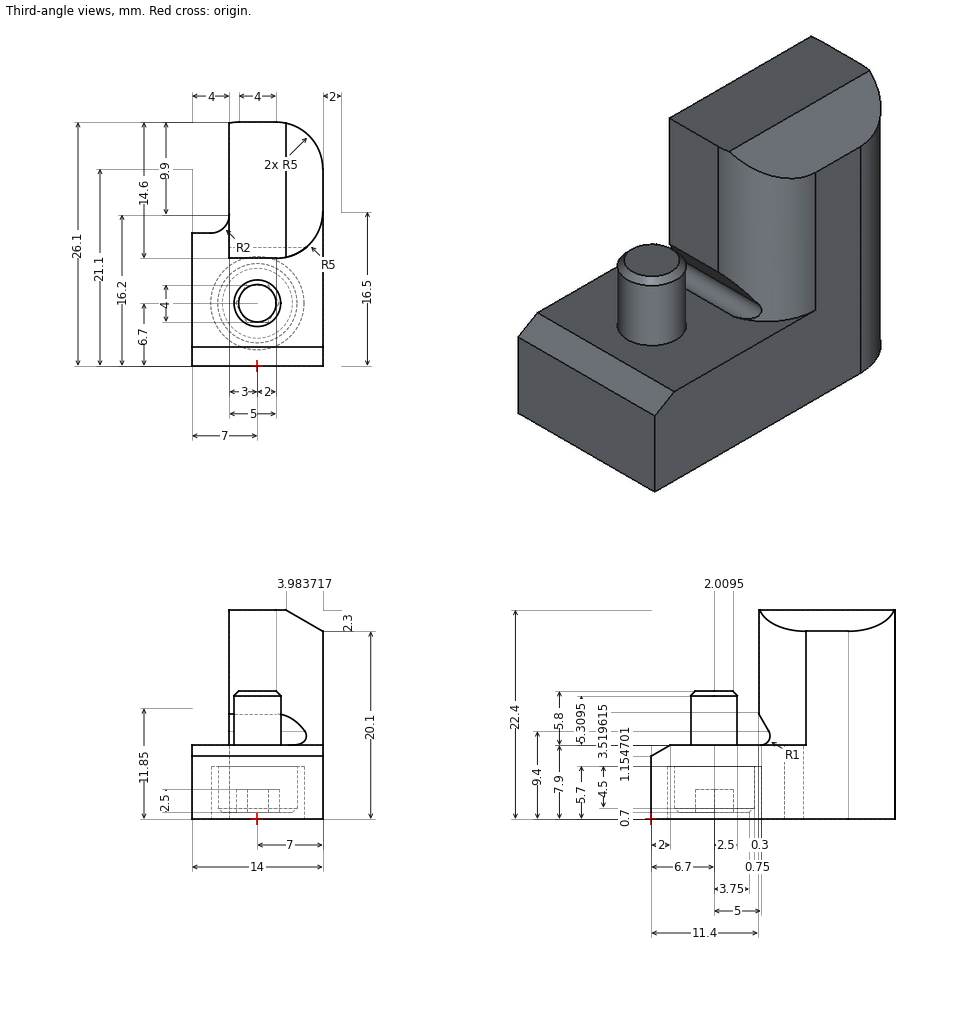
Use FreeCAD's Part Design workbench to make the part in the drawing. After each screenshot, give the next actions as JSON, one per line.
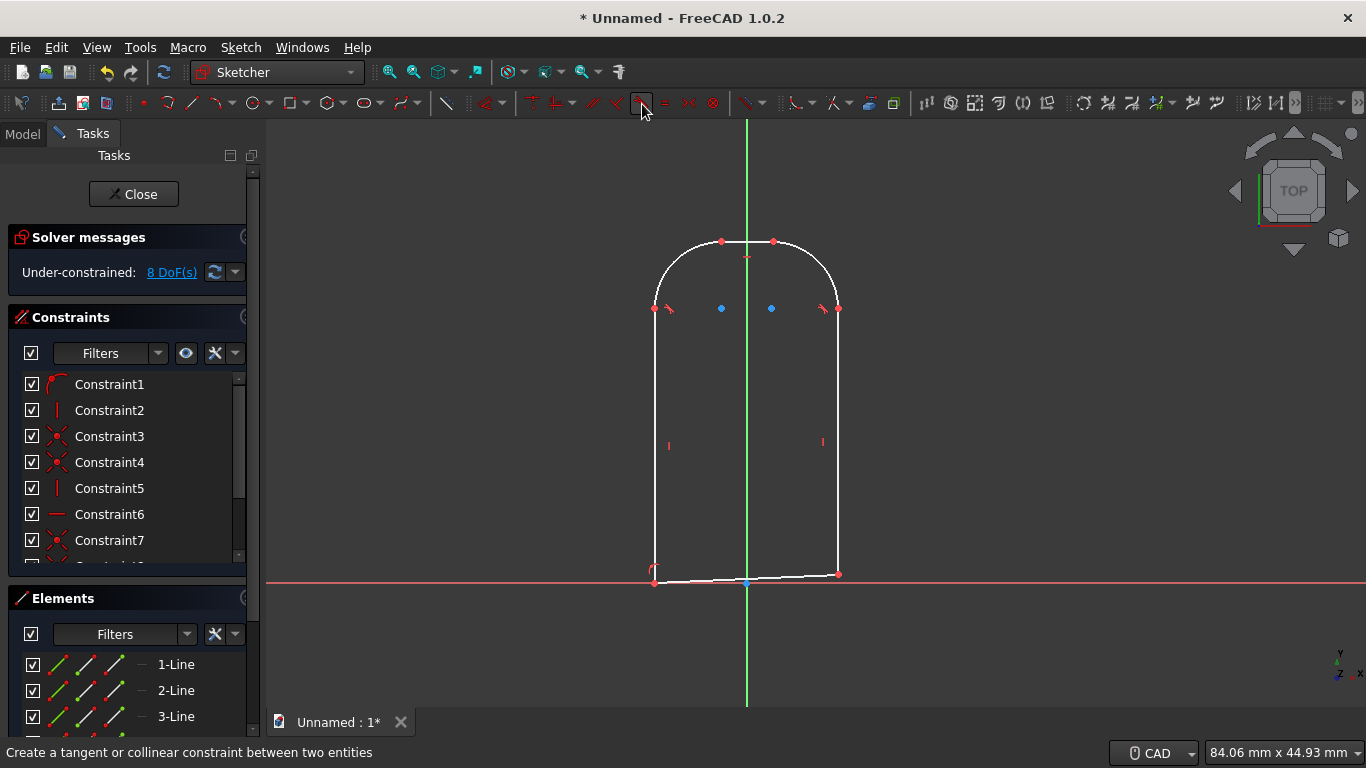
{"action": "scroll", "coordinate": [757, 242], "scroll_direction": "up", "scroll_amount": 2}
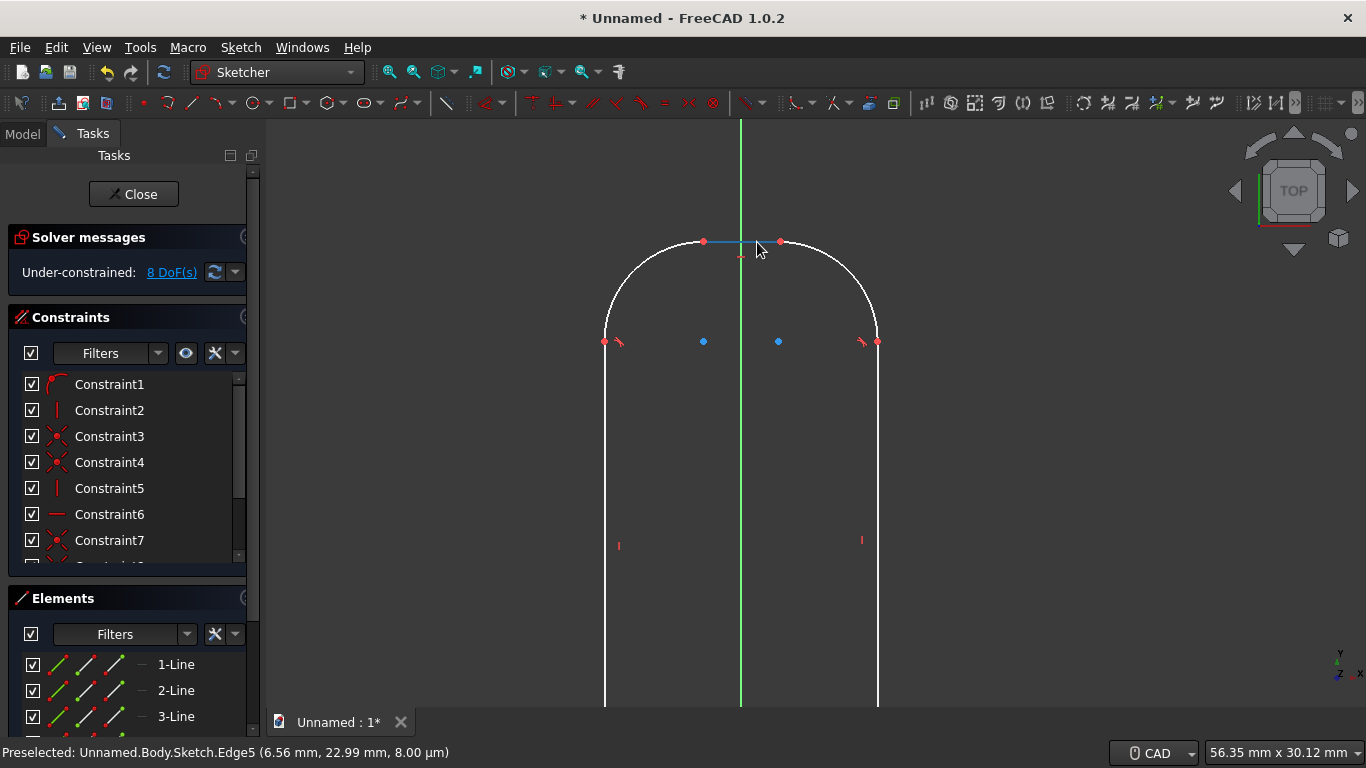
{"action": "left_click", "coordinate": [757, 242]}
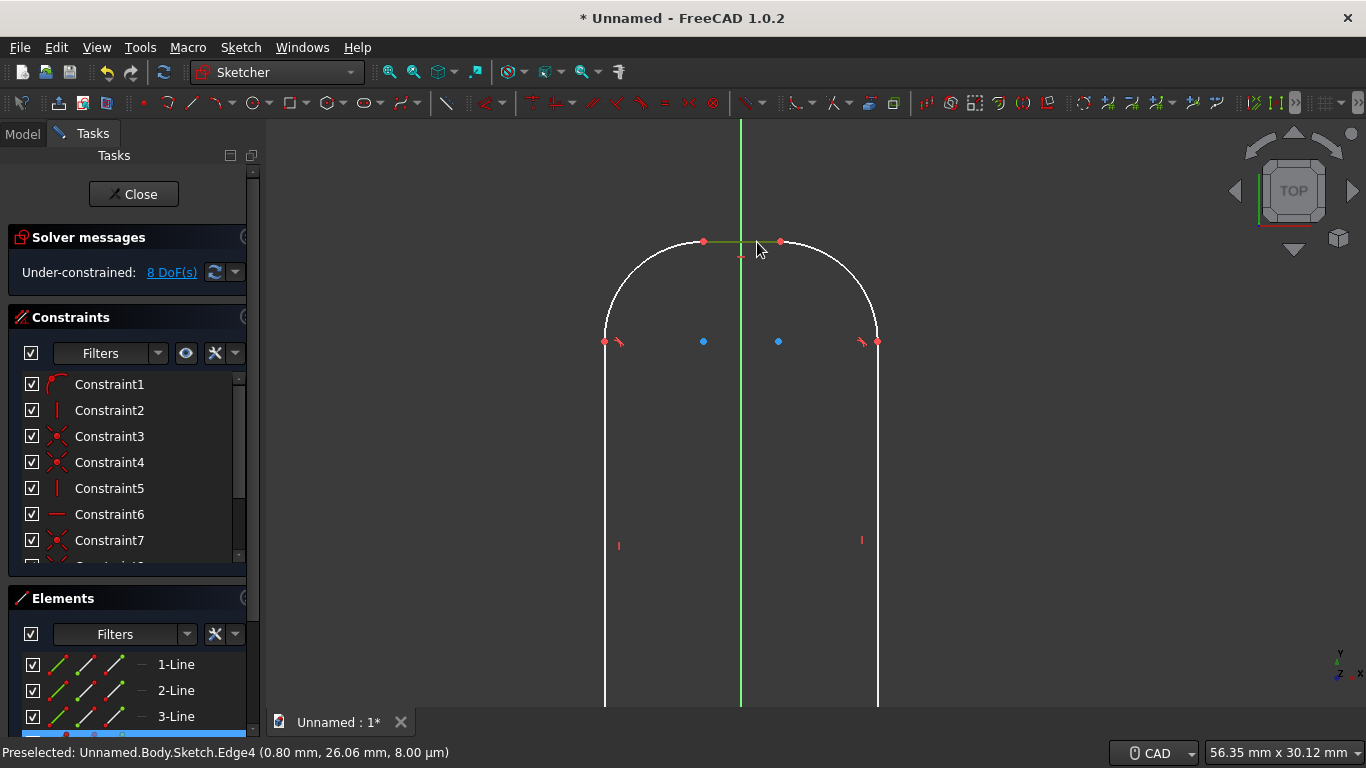
{"action": "left_click", "coordinate": [867, 297]}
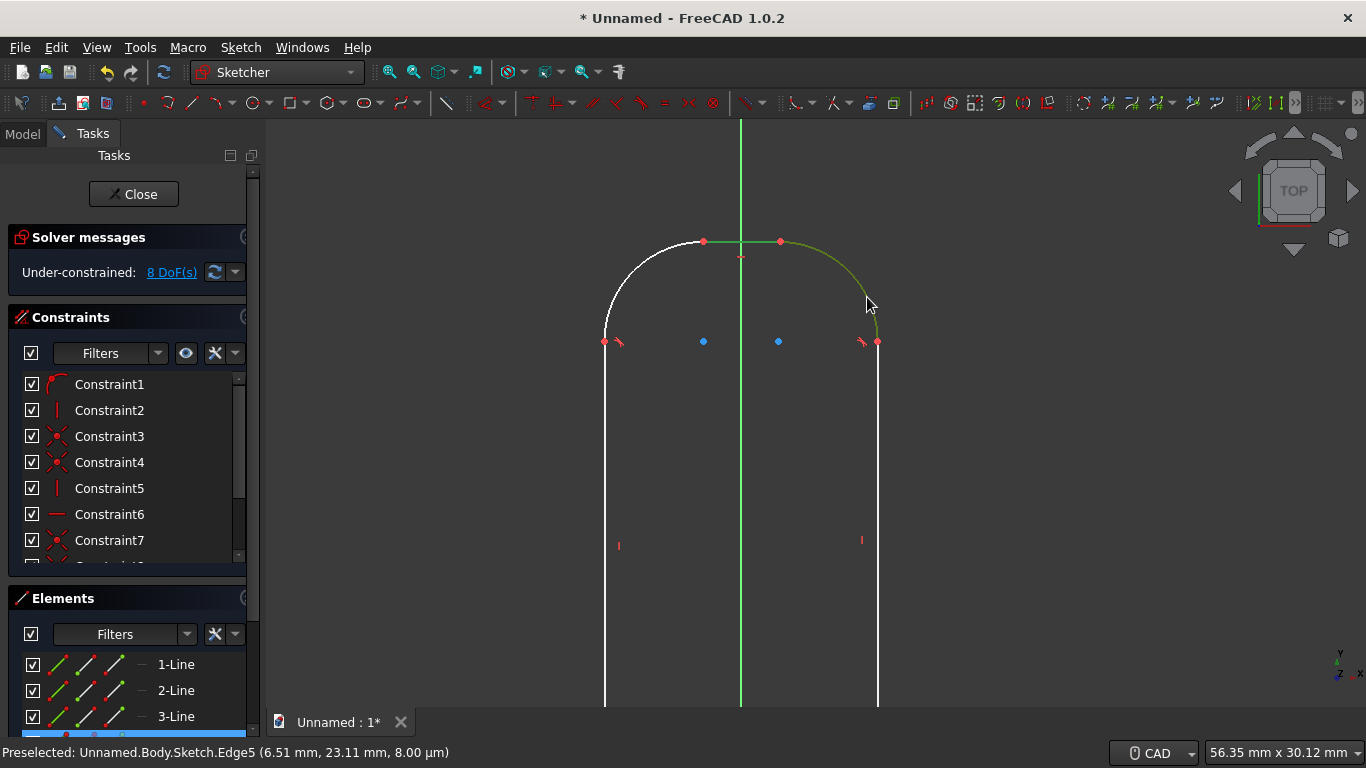
{"action": "left_click", "coordinate": [642, 104]}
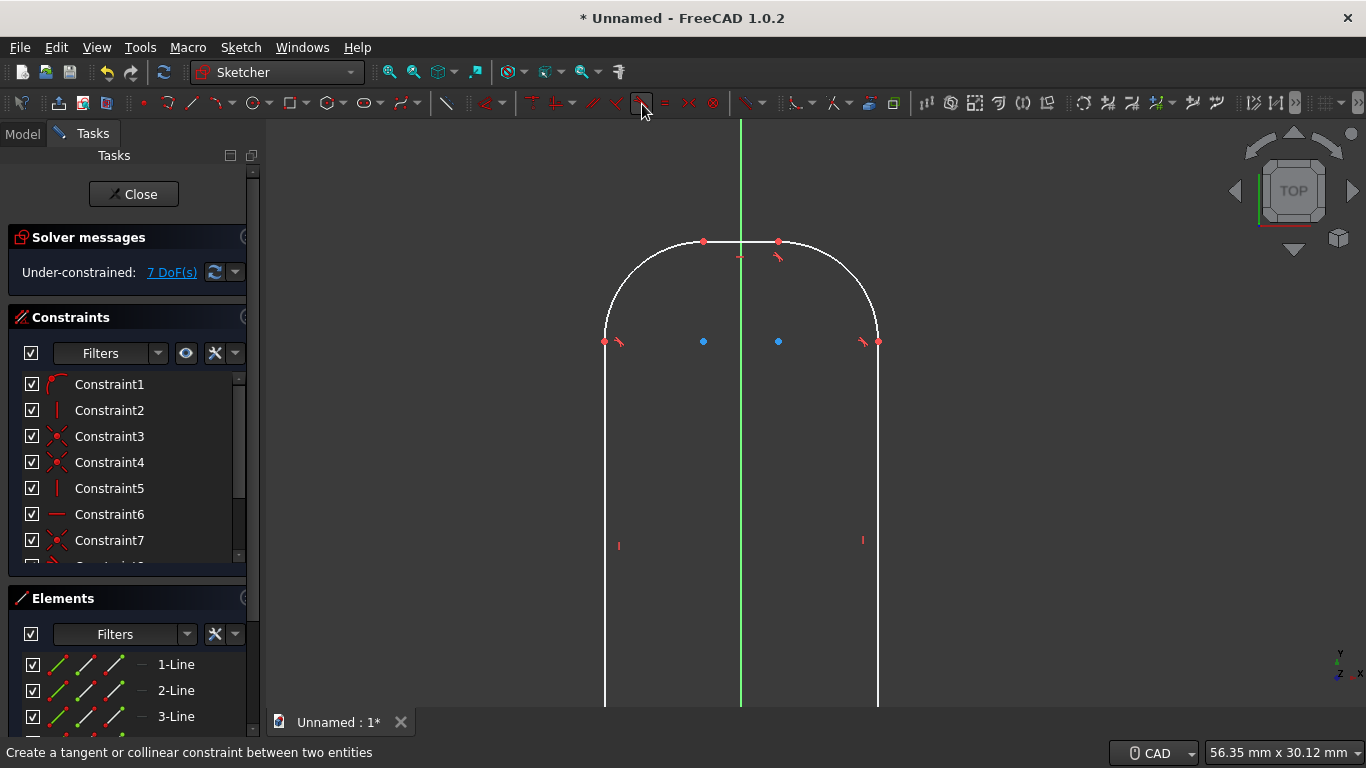
{"action": "left_click", "coordinate": [756, 242]}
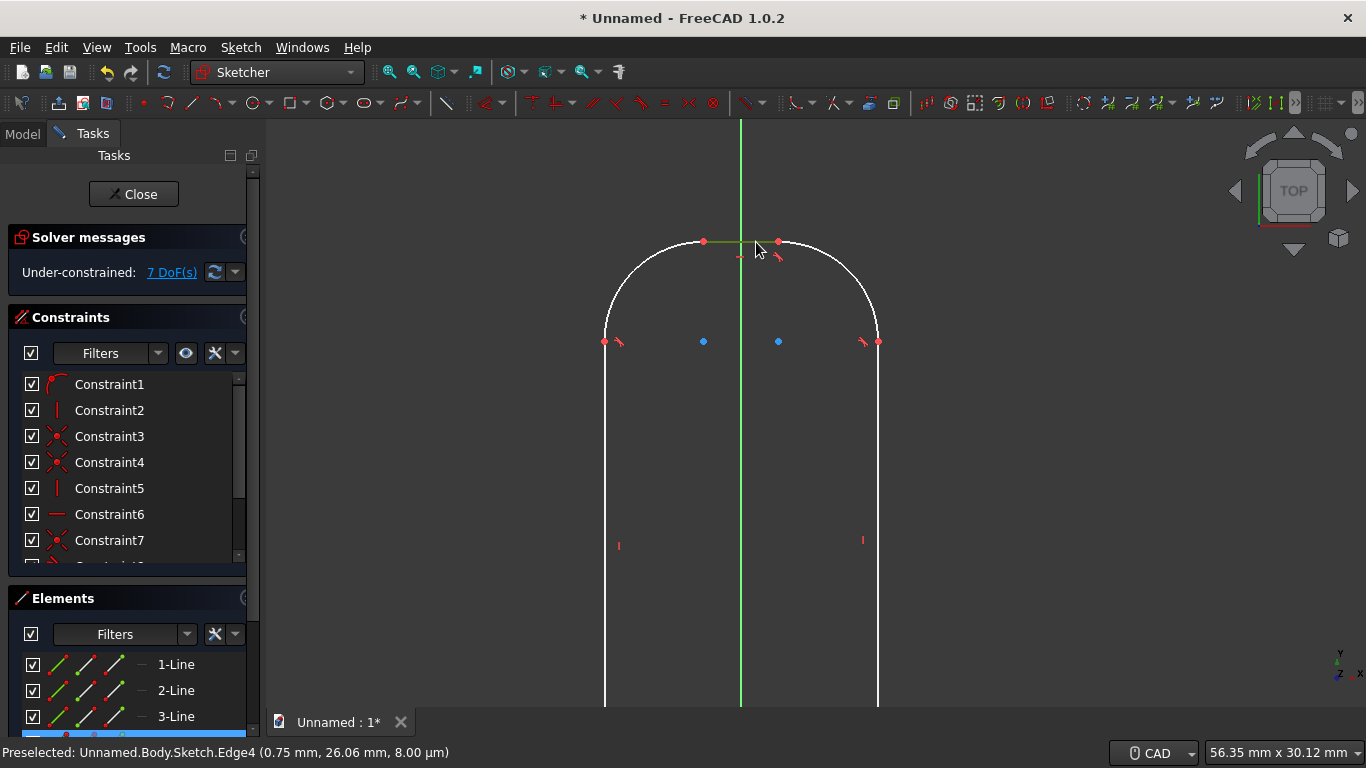
{"action": "left_click", "coordinate": [658, 253]}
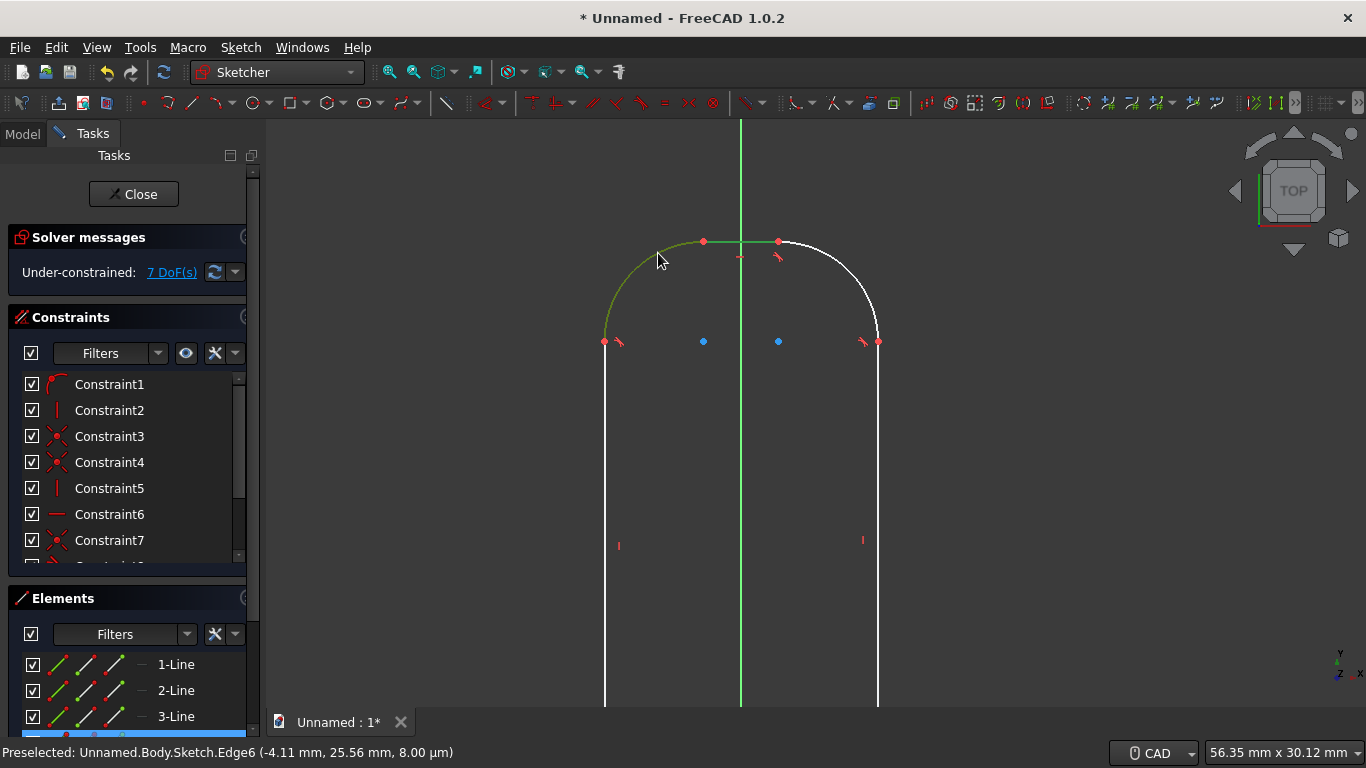
{"action": "left_click", "coordinate": [642, 104]}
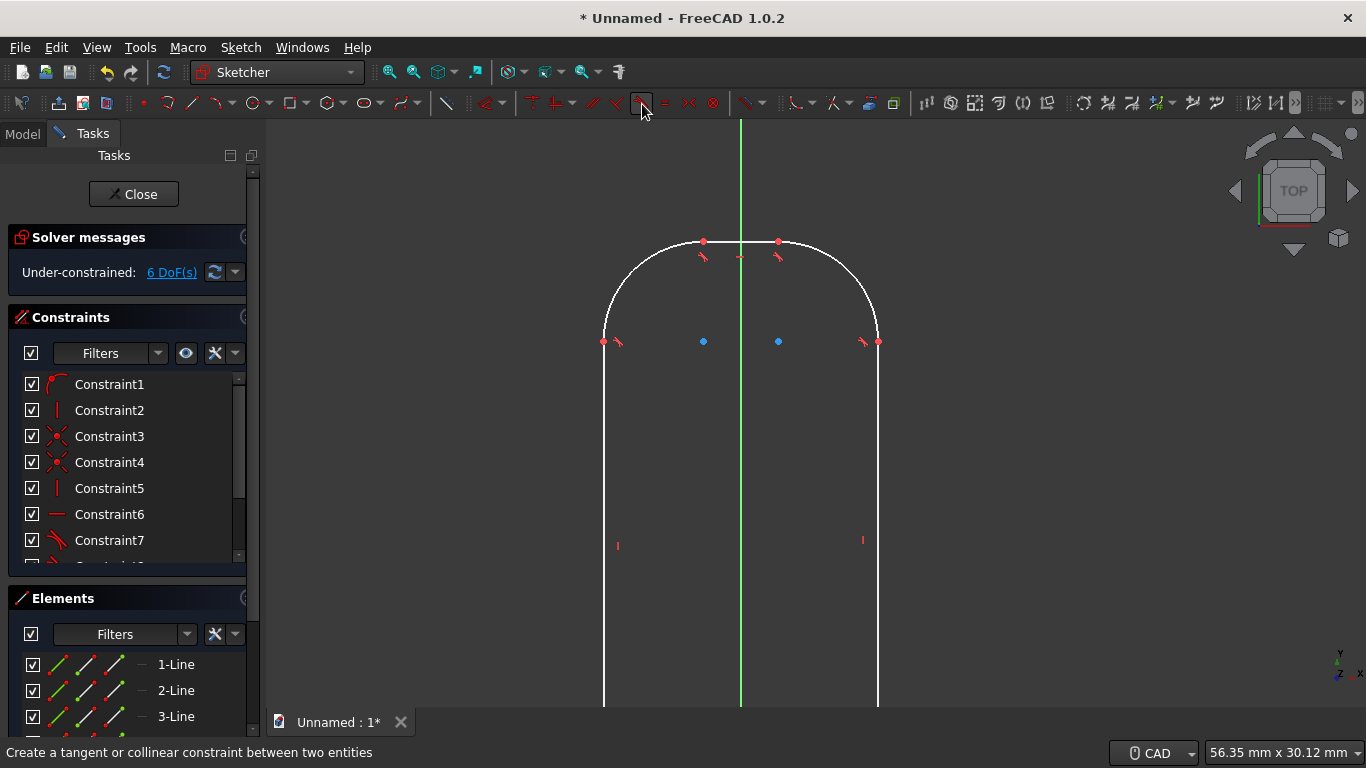
{"action": "scroll", "coordinate": [760, 244], "scroll_direction": "down", "scroll_amount": 2}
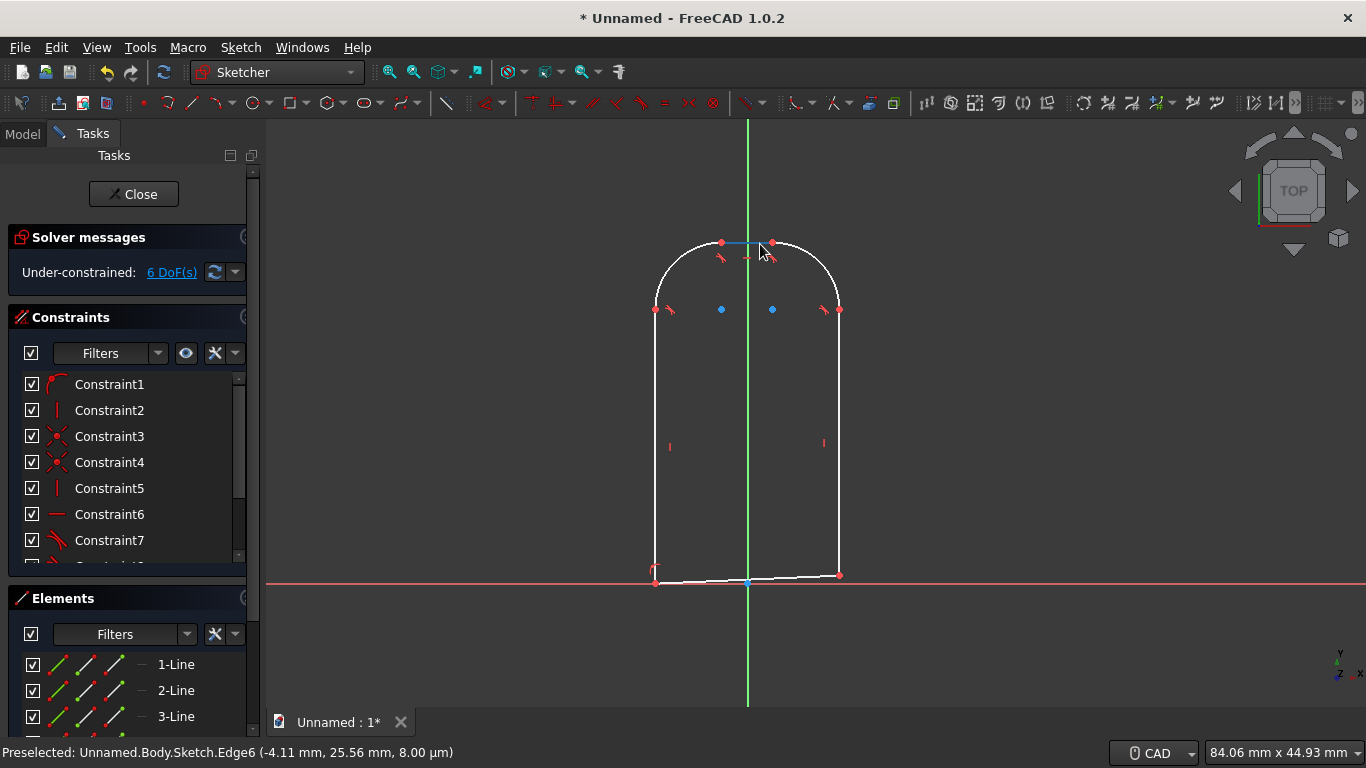
{"action": "left_click", "coordinate": [711, 581]}